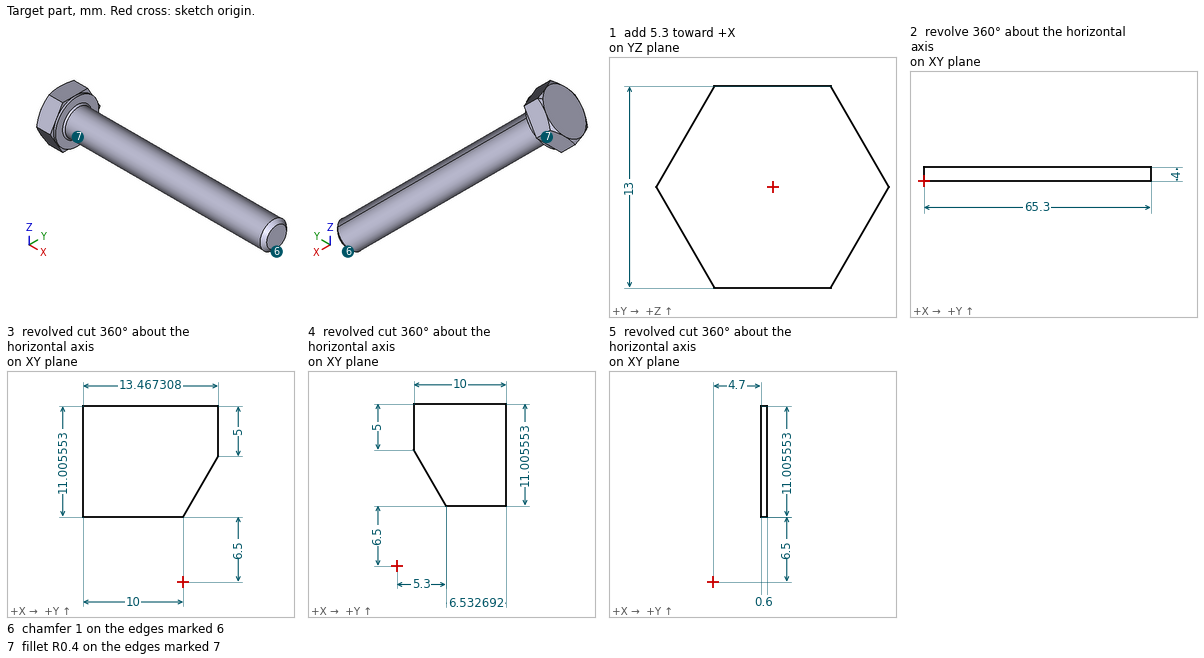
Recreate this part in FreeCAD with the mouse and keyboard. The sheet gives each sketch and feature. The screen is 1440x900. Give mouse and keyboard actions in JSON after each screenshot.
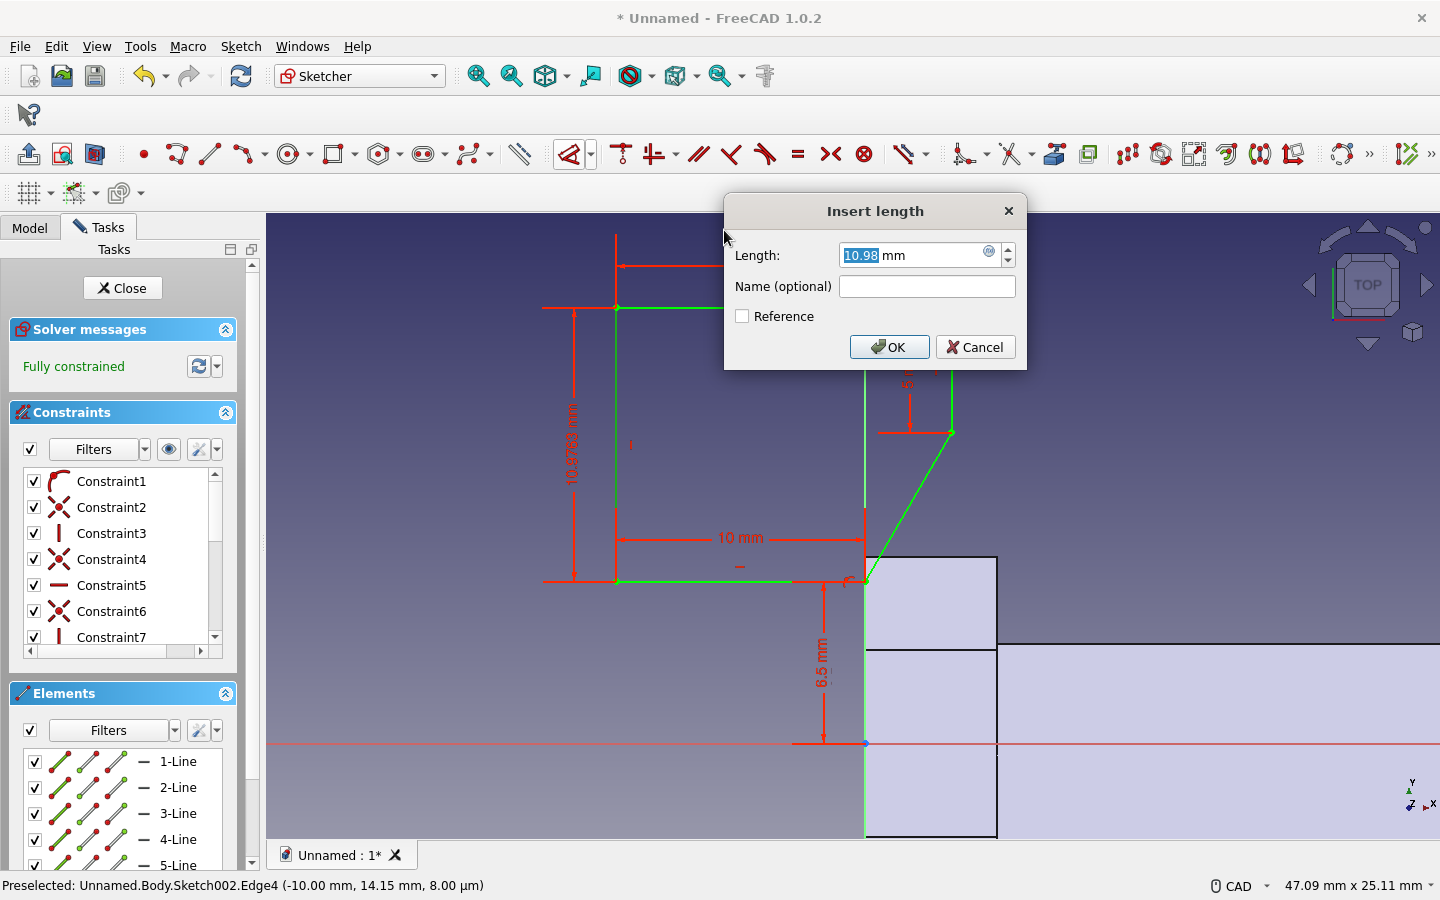
{"action": "type", "text": "11.005553"}
{"action": "key", "text": "Return"}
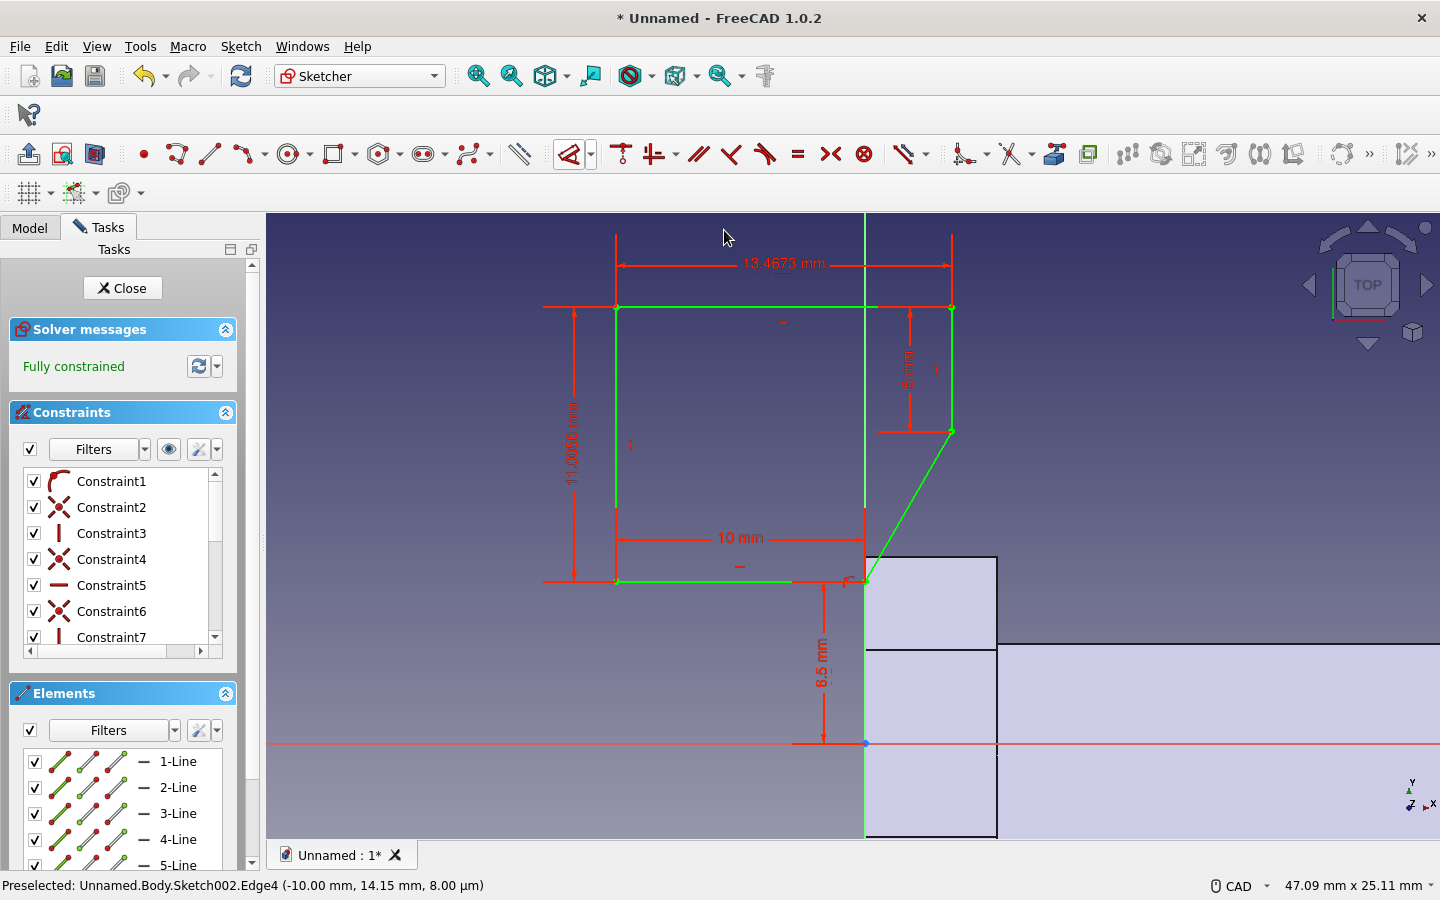
{"action": "left_click", "coordinate": [123, 288]}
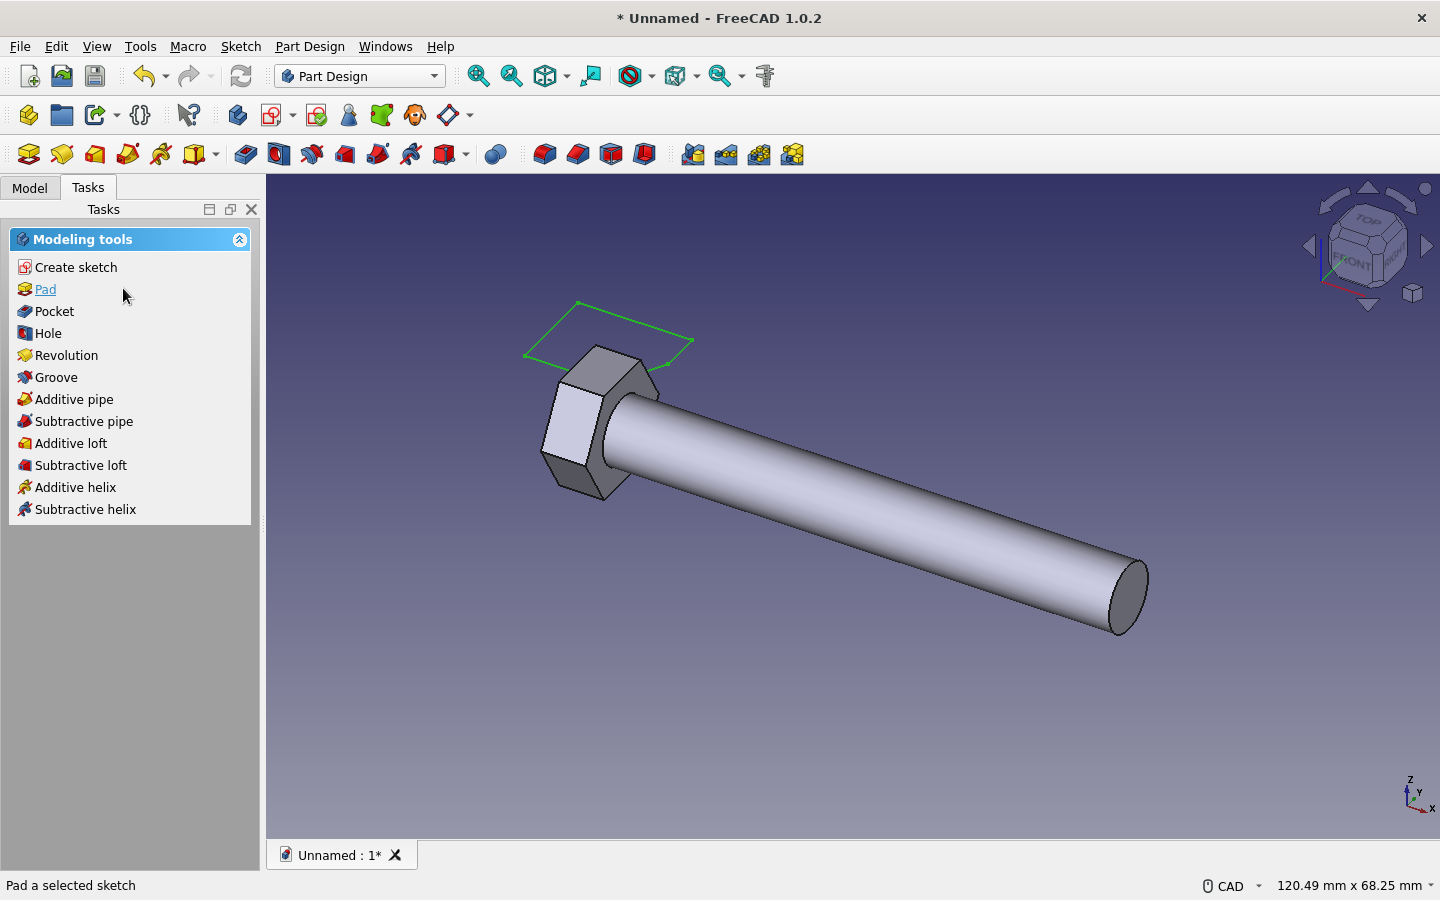
{"action": "left_click", "coordinate": [312, 154]}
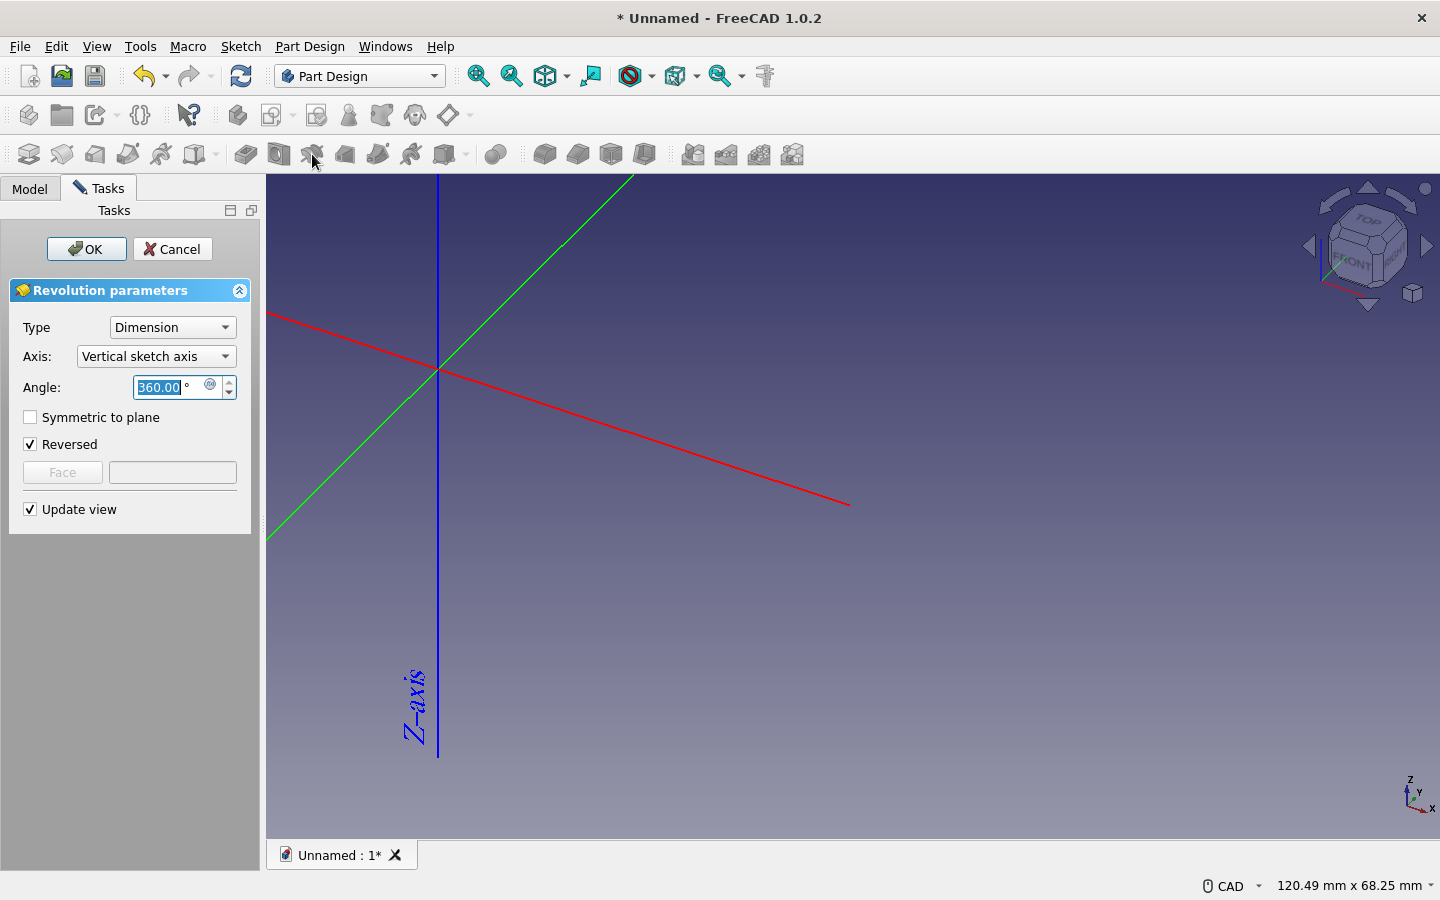
{"action": "left_click", "coordinate": [157, 356]}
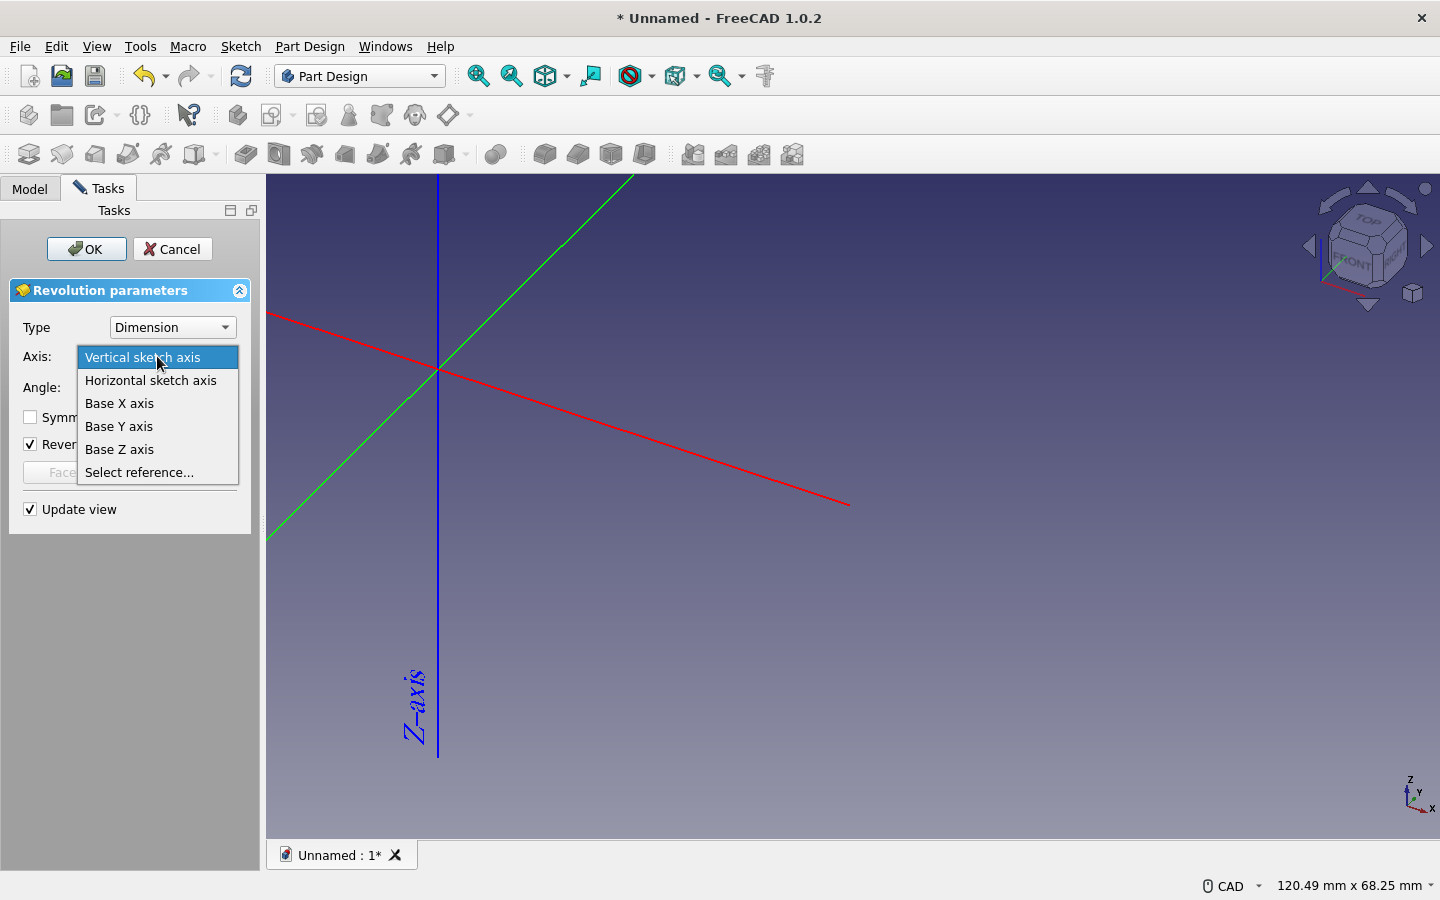
{"action": "left_click", "coordinate": [156, 380]}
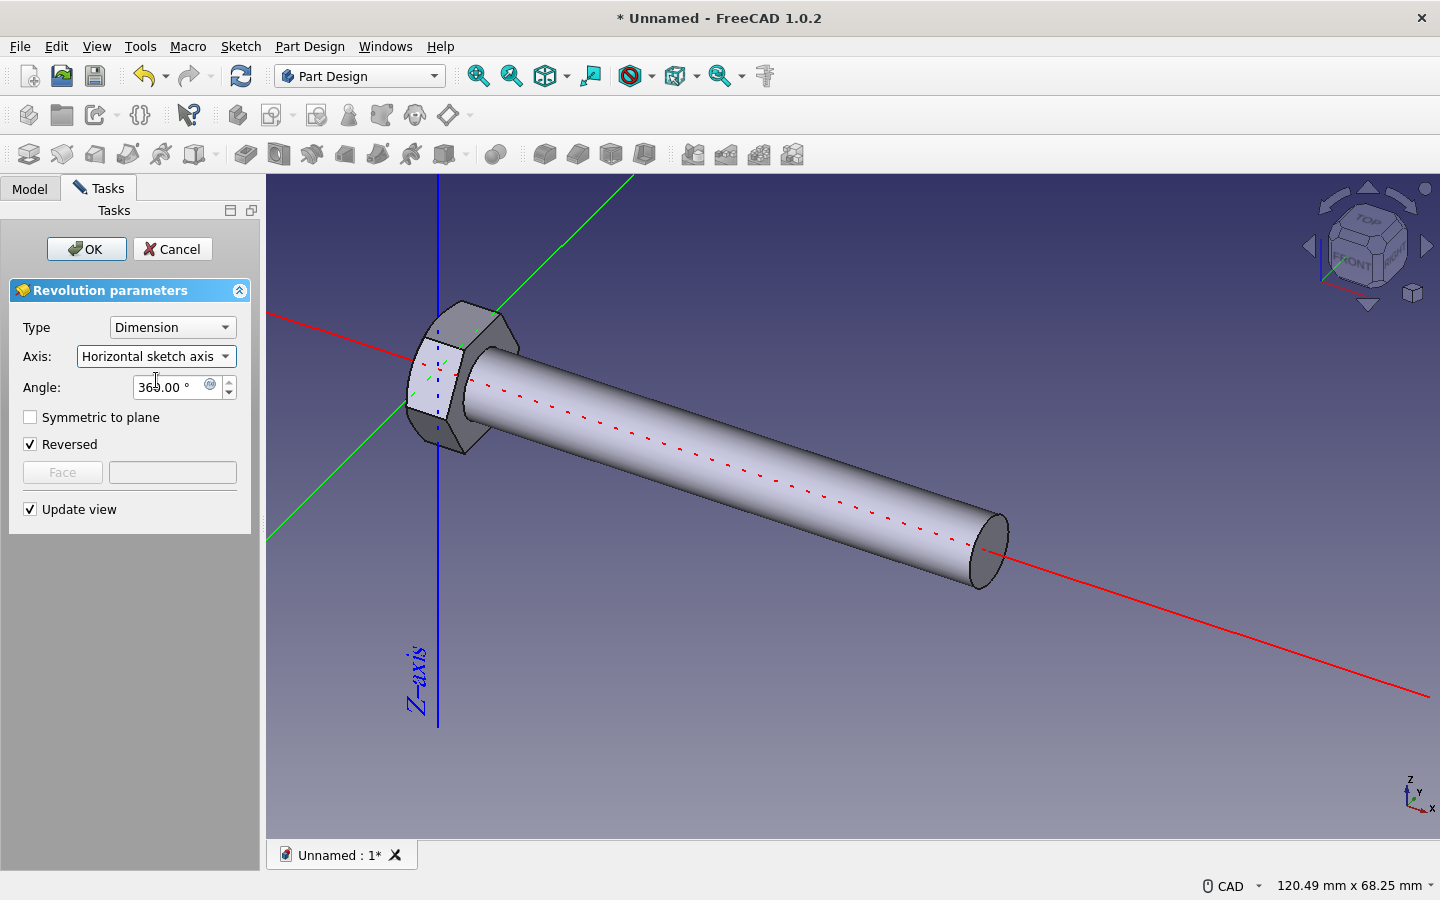
{"action": "left_click", "coordinate": [87, 249]}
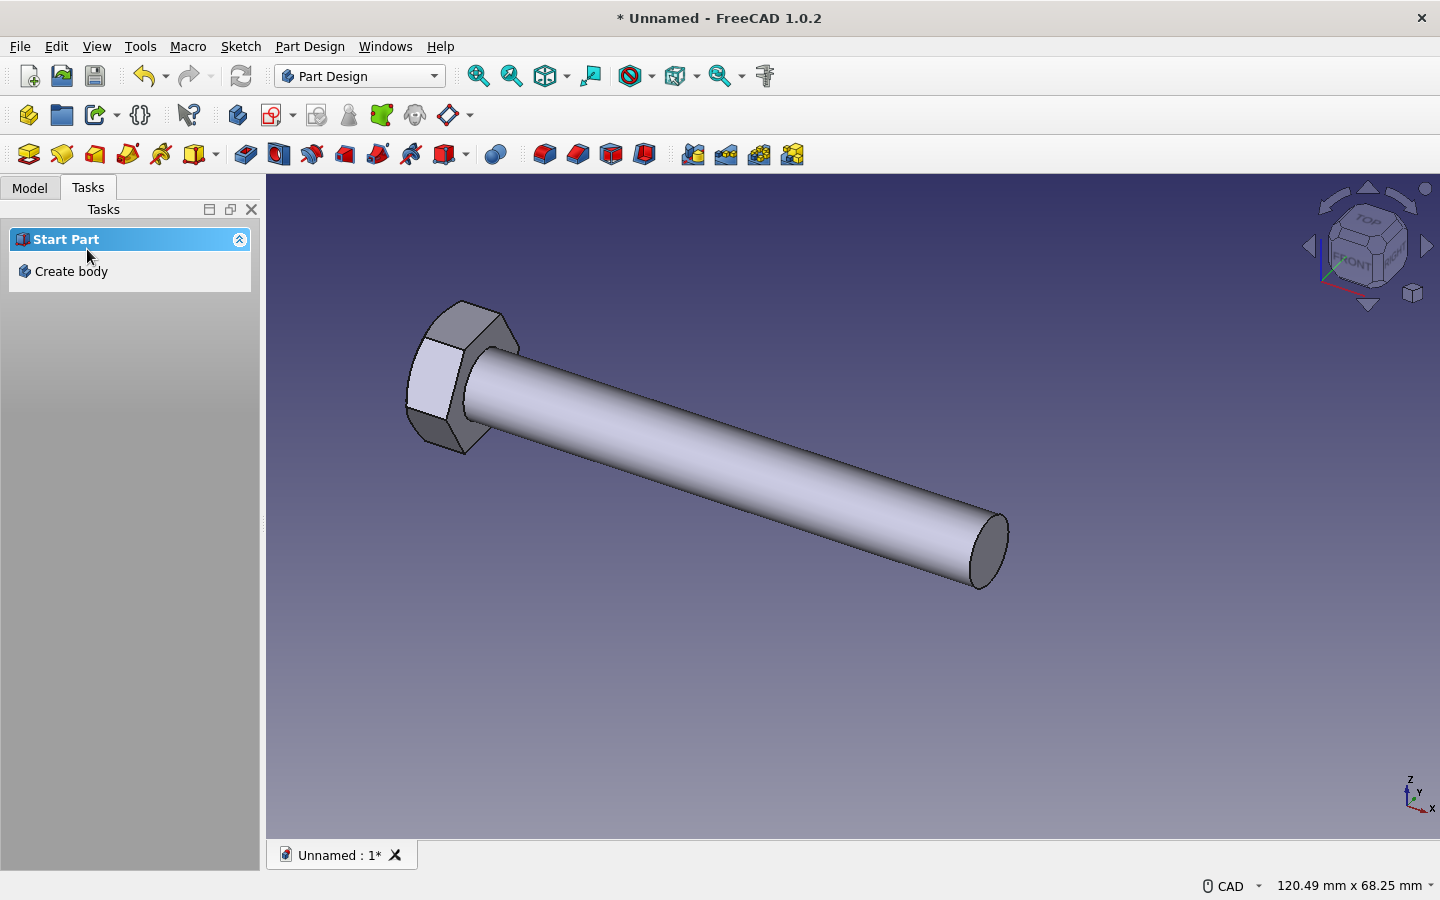
{"action": "left_click", "coordinate": [270, 116]}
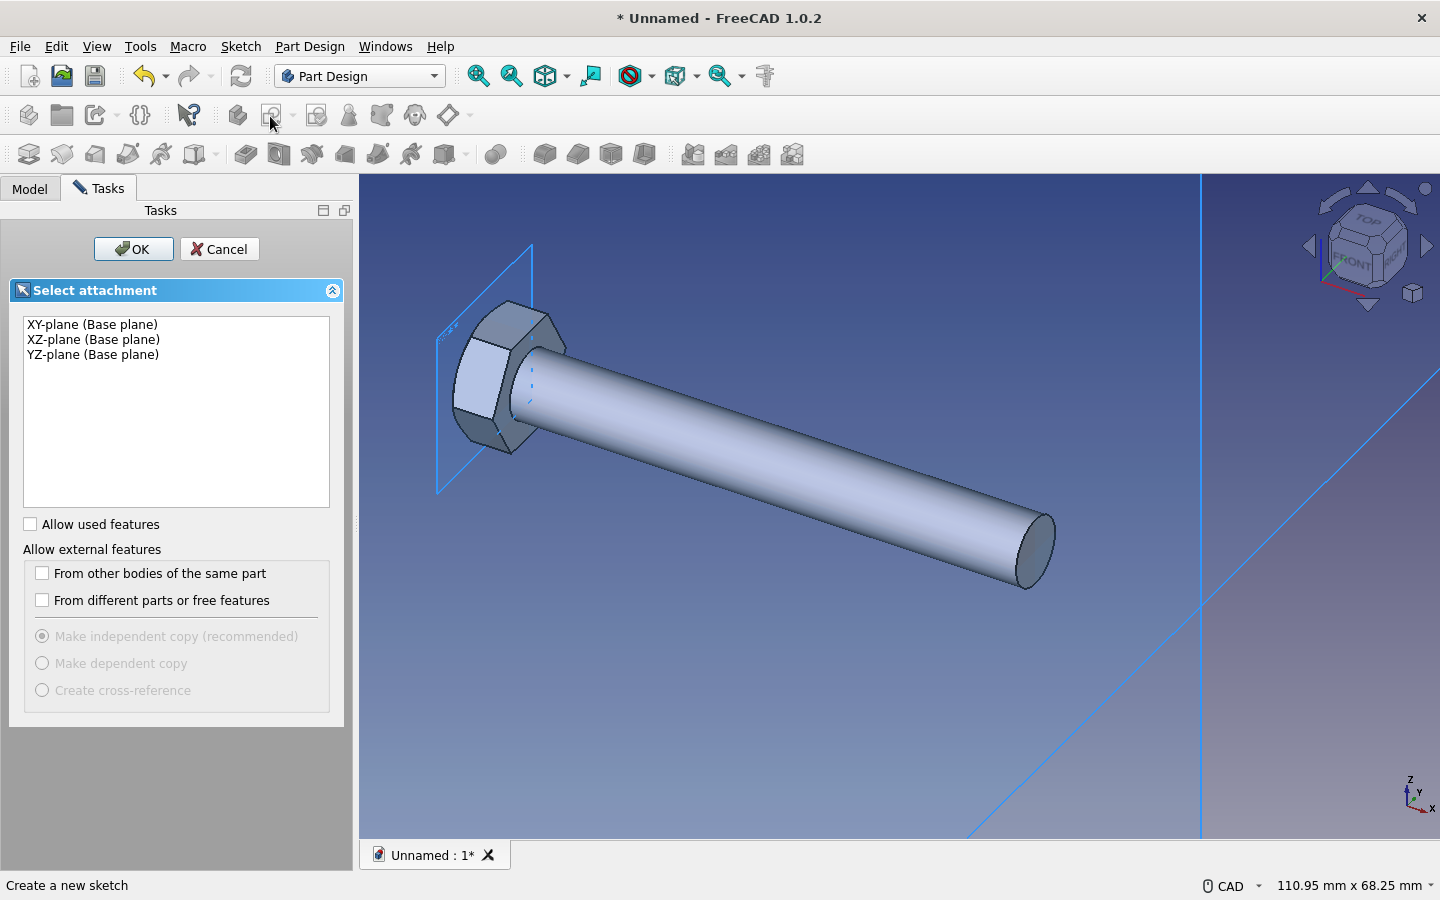
{"action": "left_click", "coordinate": [84, 324]}